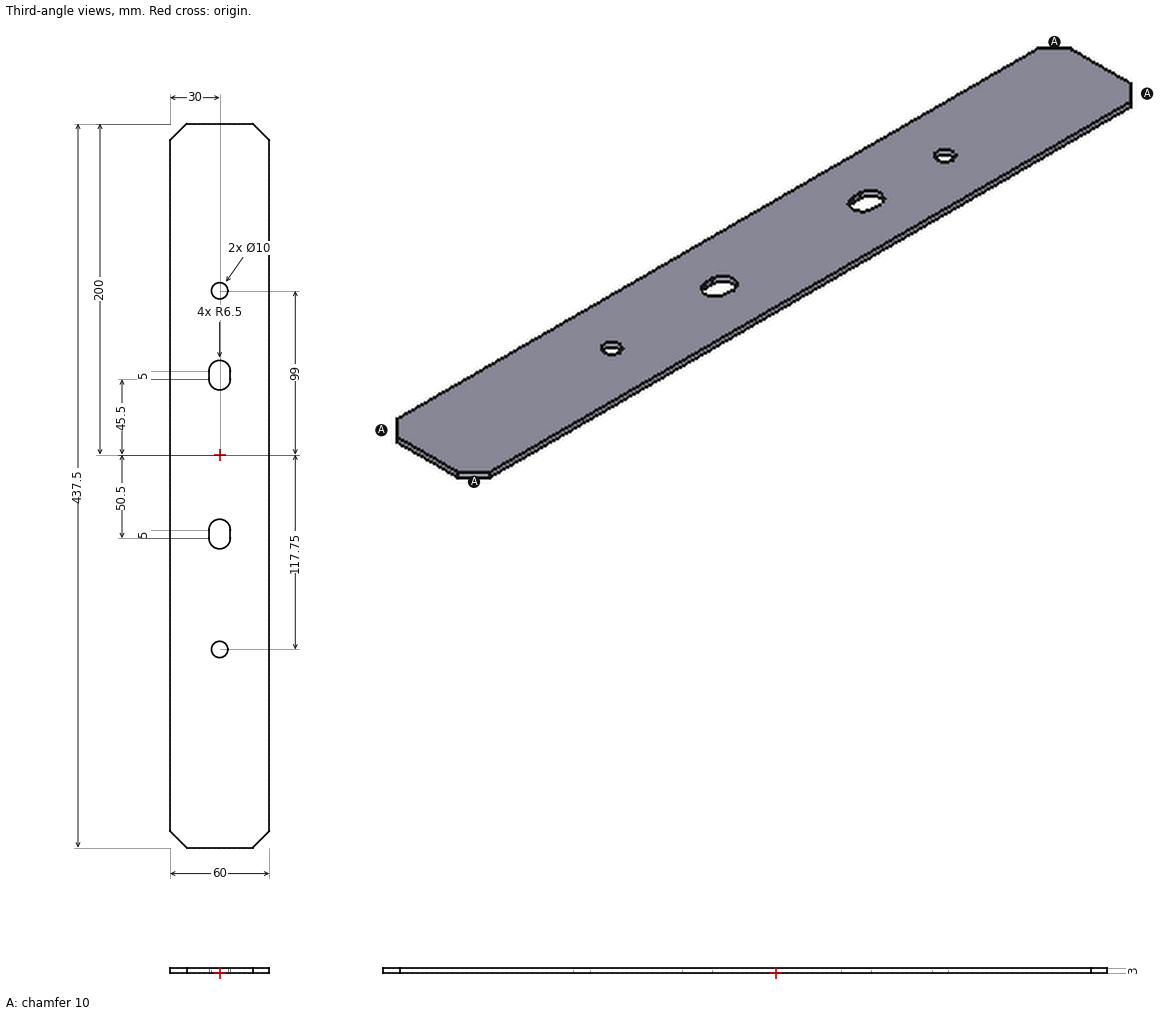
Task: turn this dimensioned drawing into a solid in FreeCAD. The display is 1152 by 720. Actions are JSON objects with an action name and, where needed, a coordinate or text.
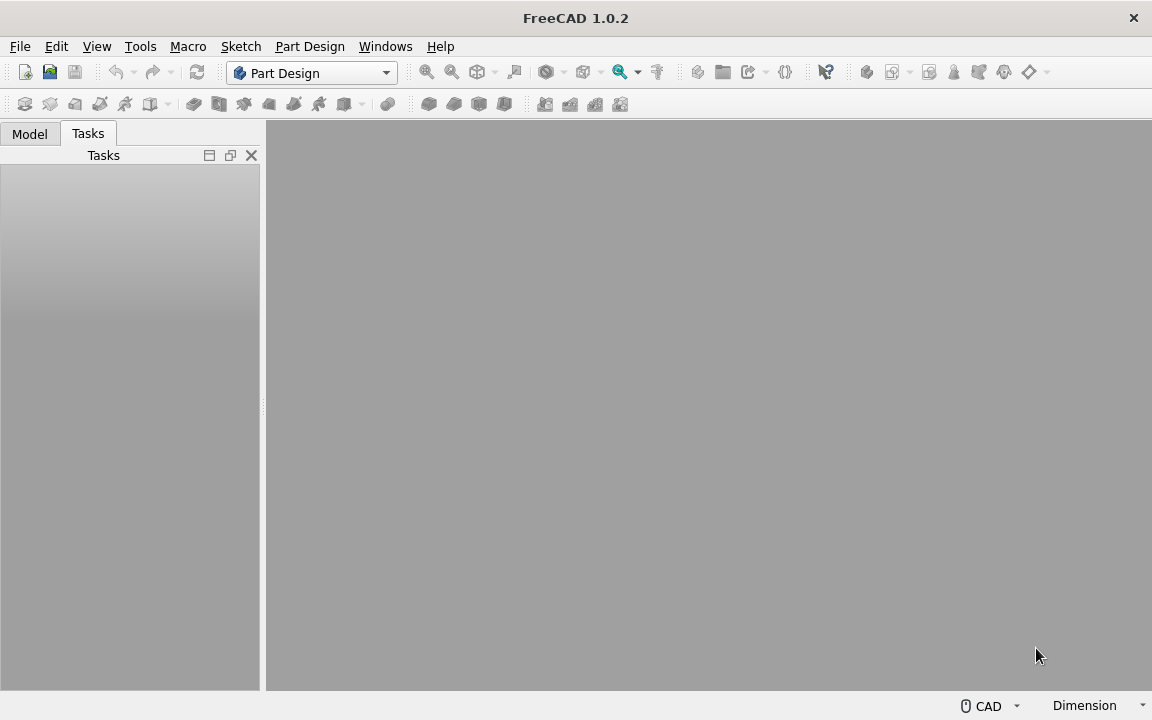
{"action": "left_click", "coordinate": [25, 72]}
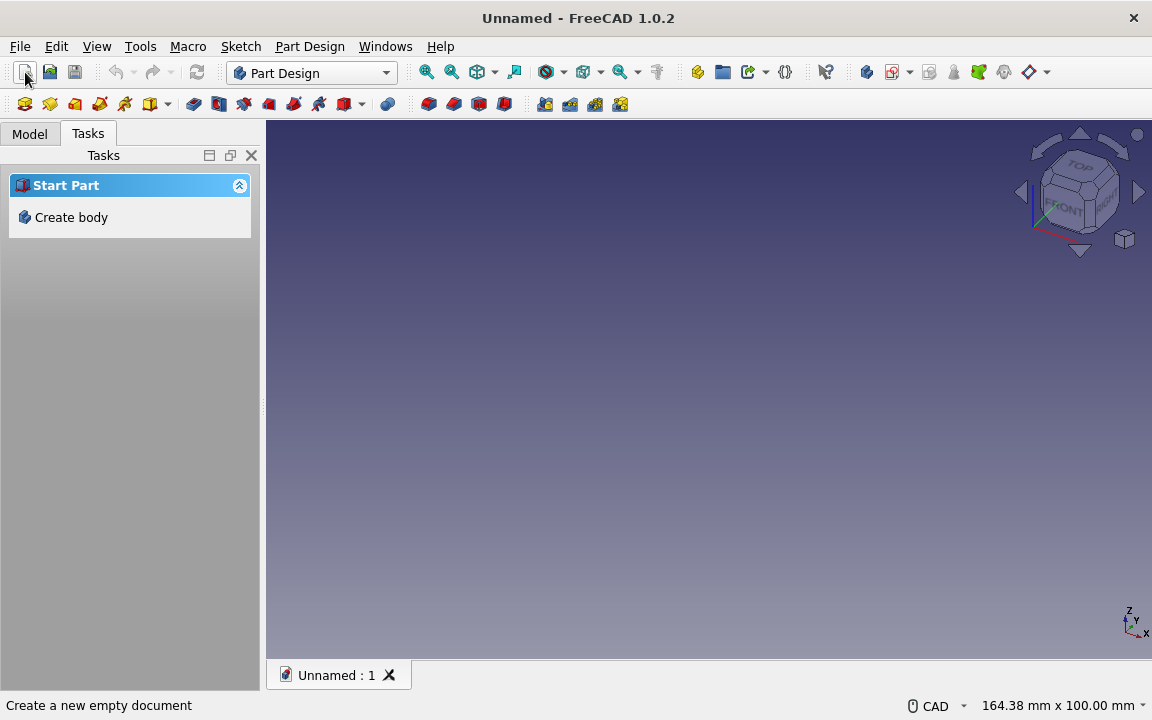
{"action": "left_click", "coordinate": [892, 72]}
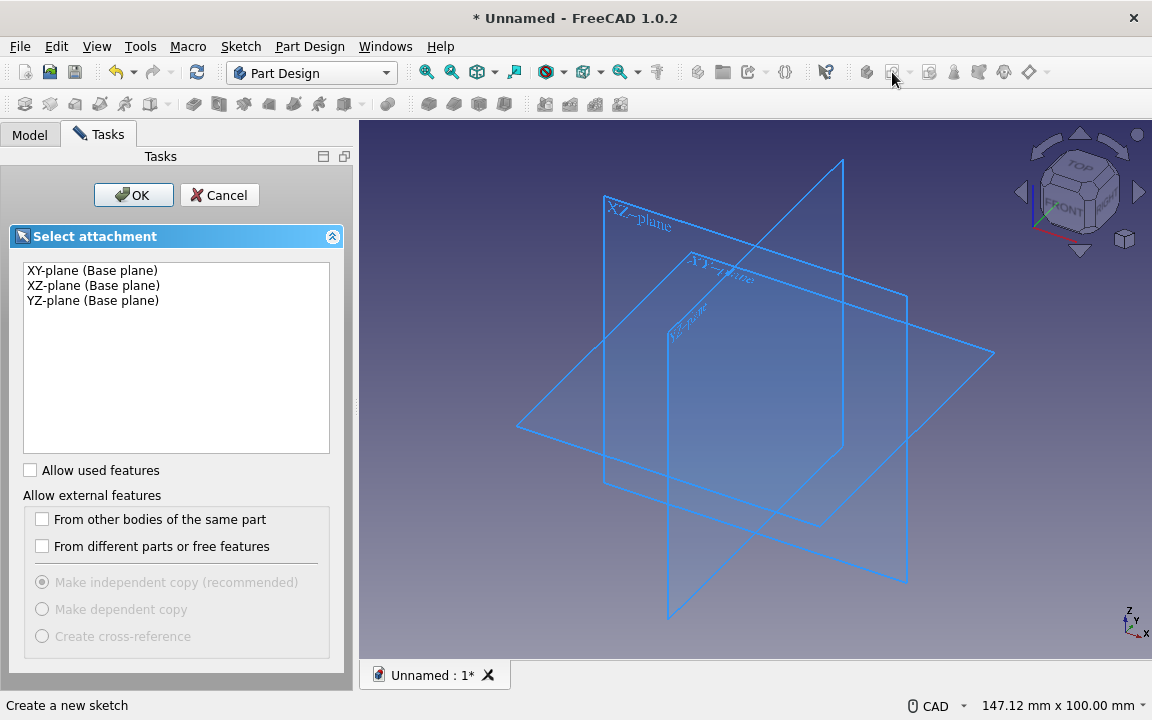
{"action": "left_click", "coordinate": [84, 270]}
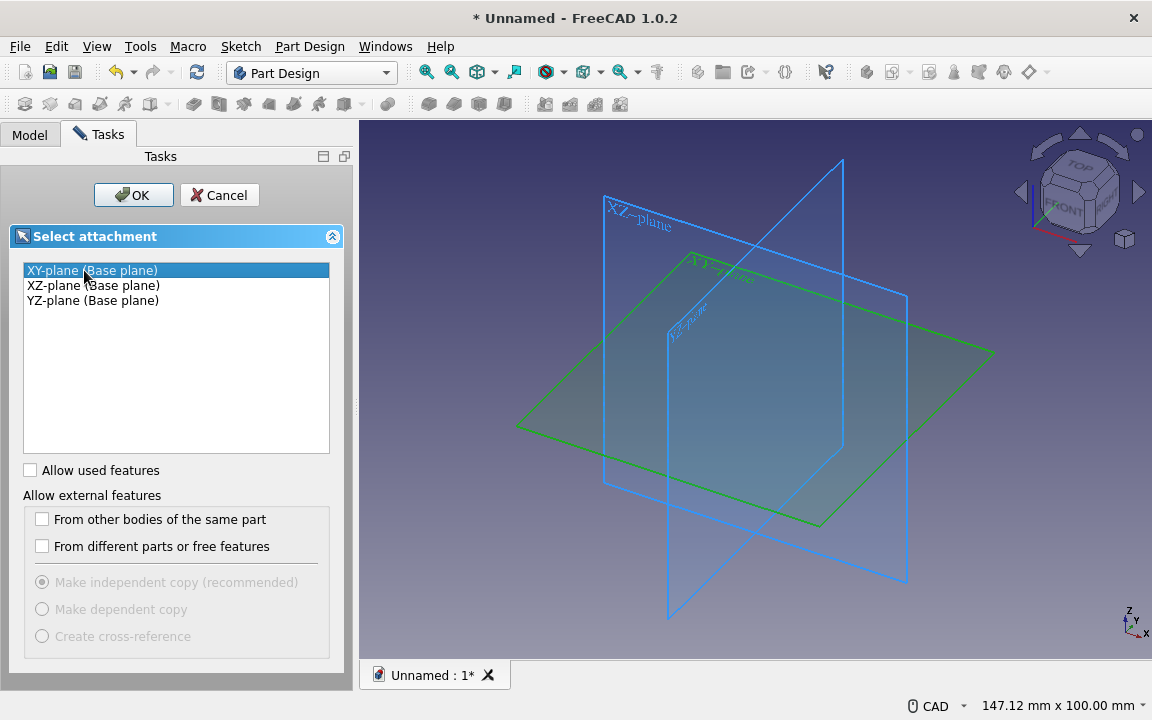
{"action": "left_click", "coordinate": [134, 195]}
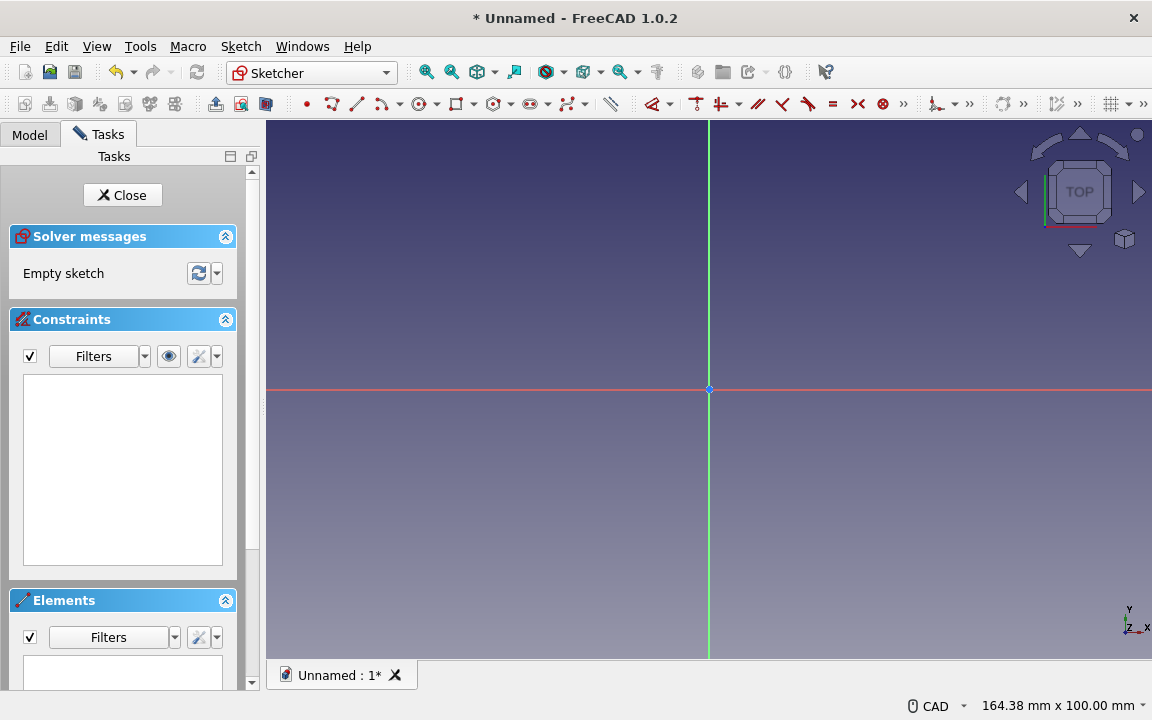
{"action": "scroll", "coordinate": [630, 374], "scroll_direction": "down", "scroll_amount": 10}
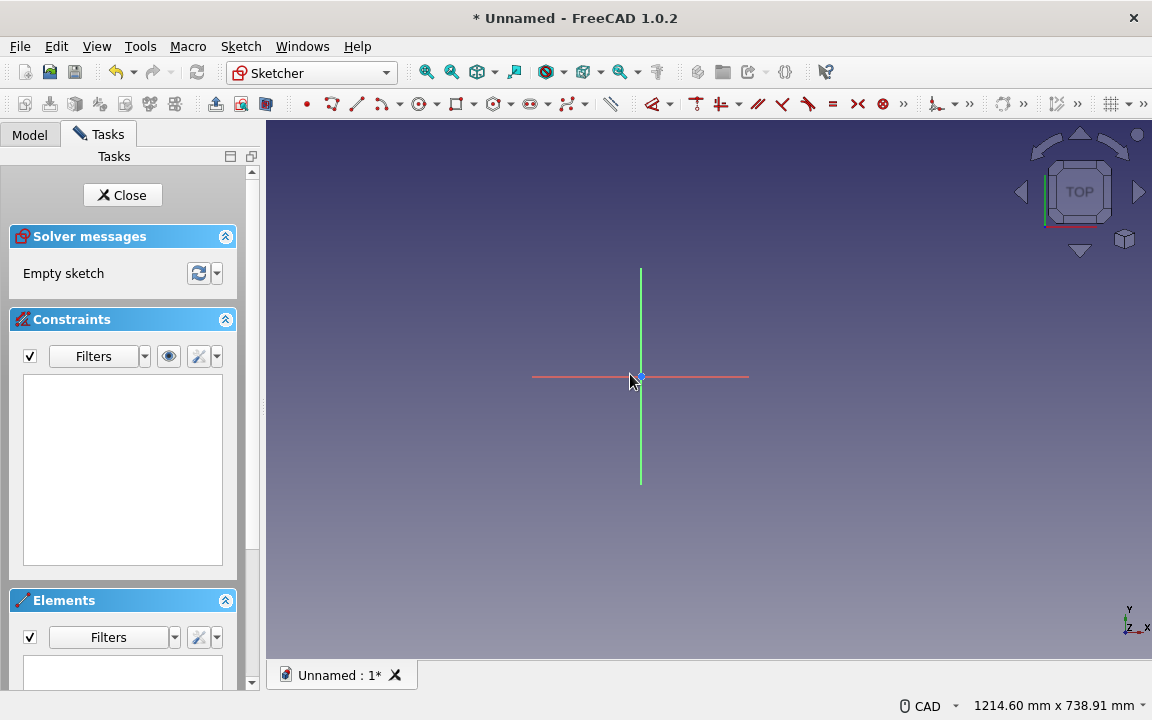
{"action": "left_click", "coordinate": [456, 104]}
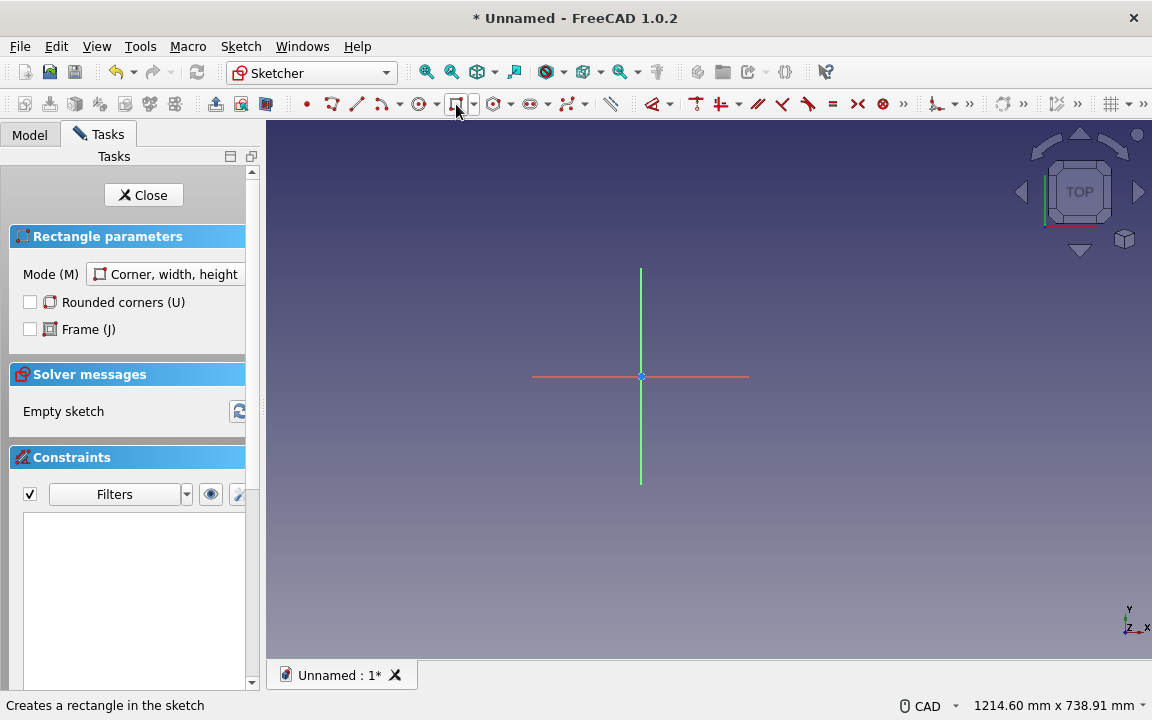
{"action": "left_click", "coordinate": [619, 231]}
{"action": "left_click", "coordinate": [663, 550]}
{"action": "key", "text": "Escape"}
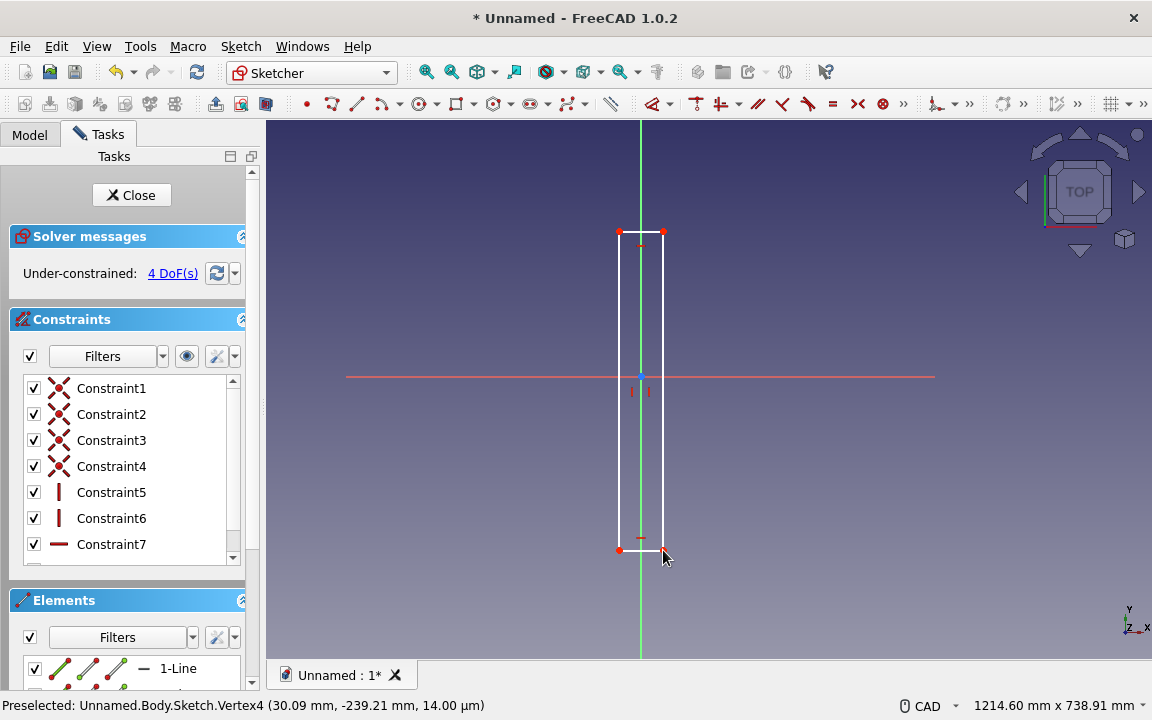
{"action": "left_click", "coordinate": [652, 104]}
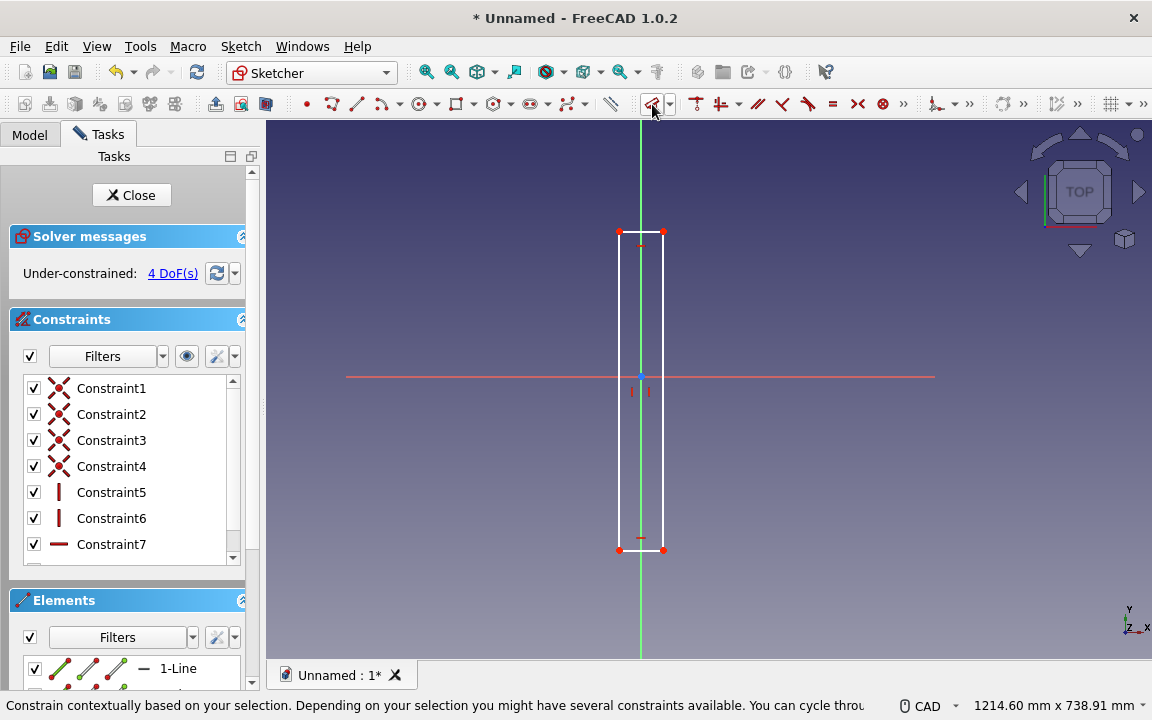
{"action": "left_click", "coordinate": [641, 551]}
{"action": "left_click", "coordinate": [626, 585]}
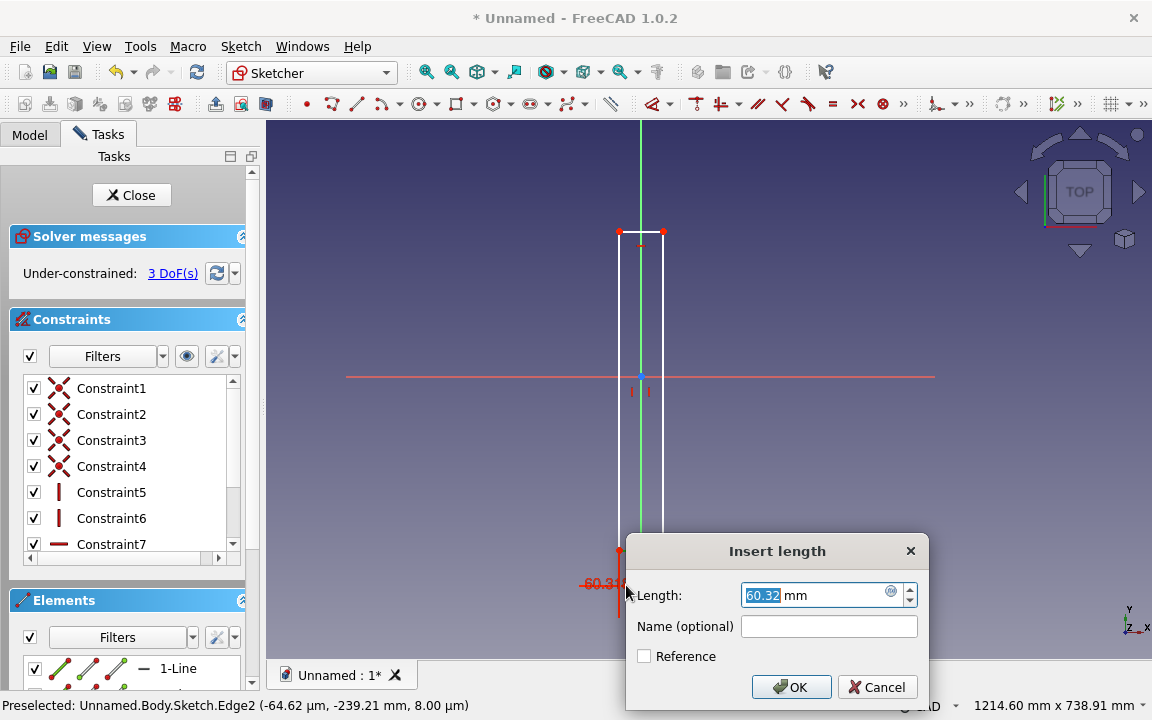
{"action": "type", "text": "60"}
{"action": "key", "text": "Return"}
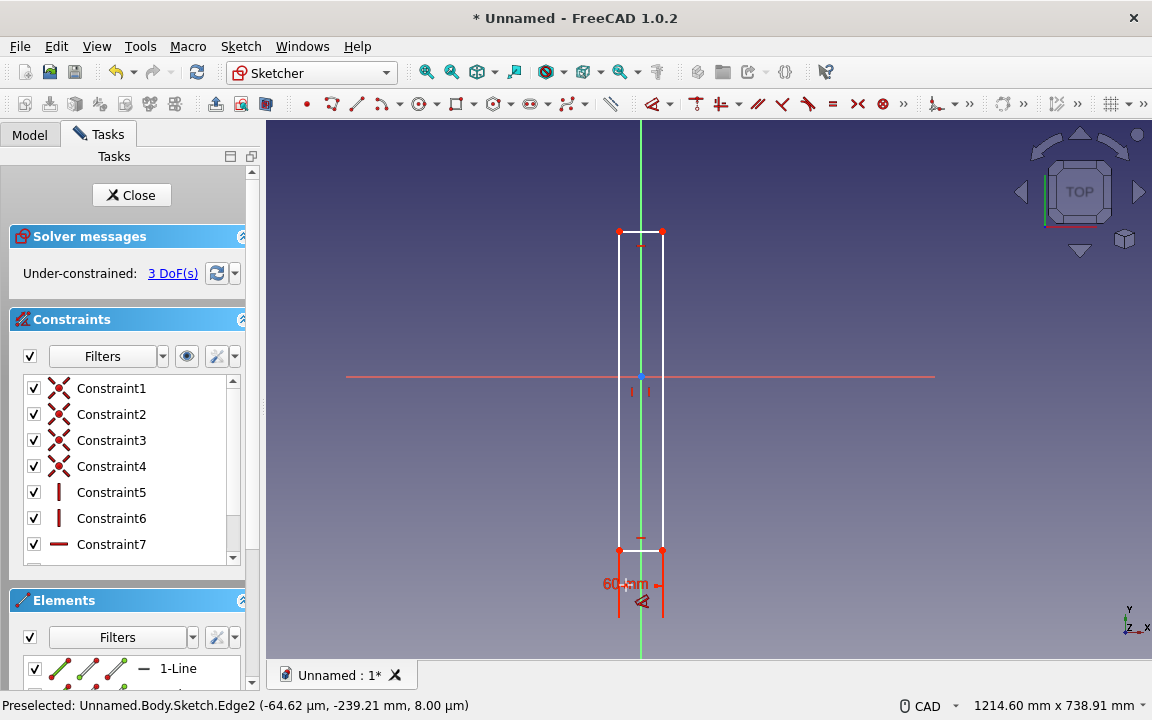
{"action": "scroll", "coordinate": [619, 232], "scroll_direction": "up", "scroll_amount": 3}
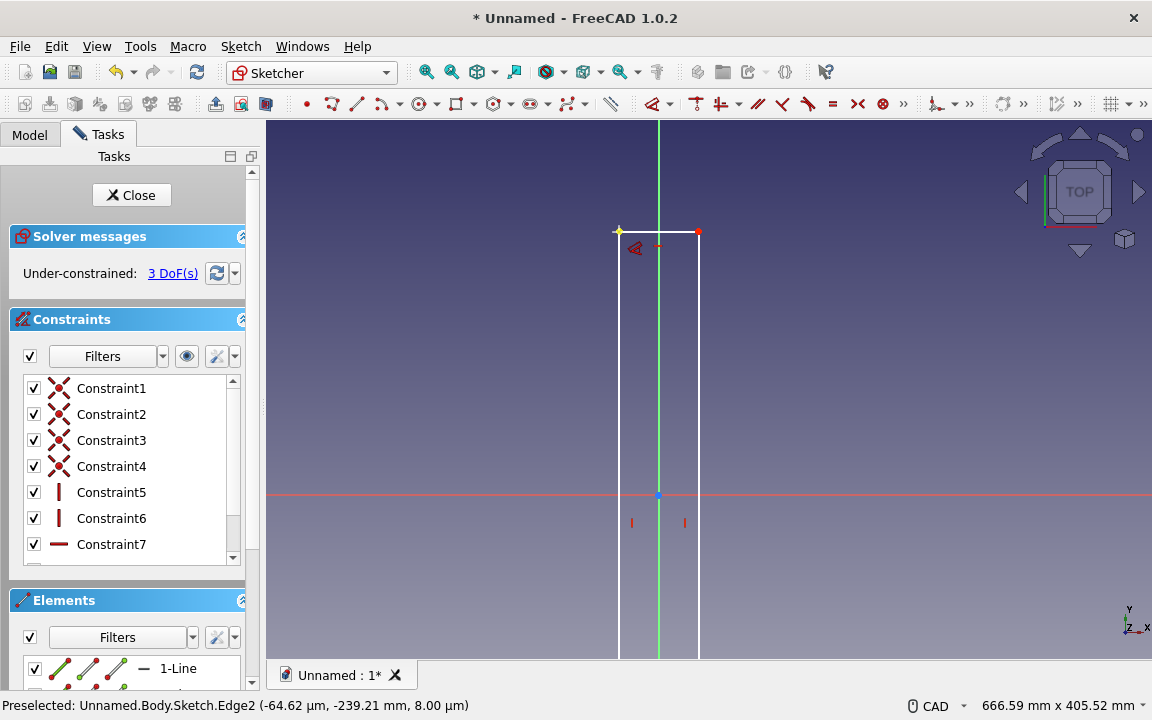
{"action": "left_click", "coordinate": [619, 232]}
{"action": "left_click", "coordinate": [639, 198]}